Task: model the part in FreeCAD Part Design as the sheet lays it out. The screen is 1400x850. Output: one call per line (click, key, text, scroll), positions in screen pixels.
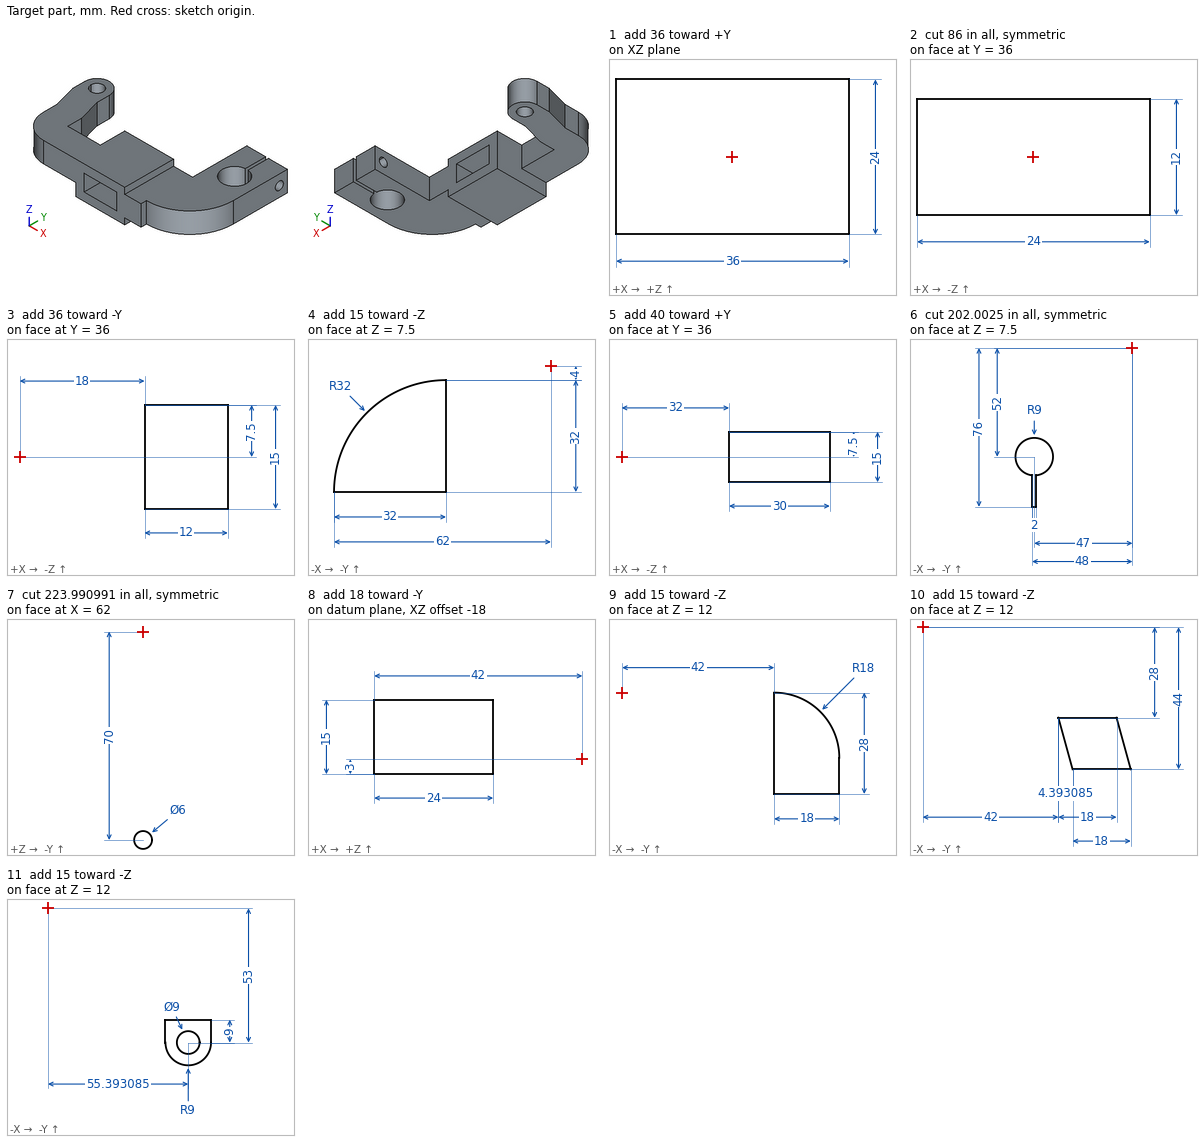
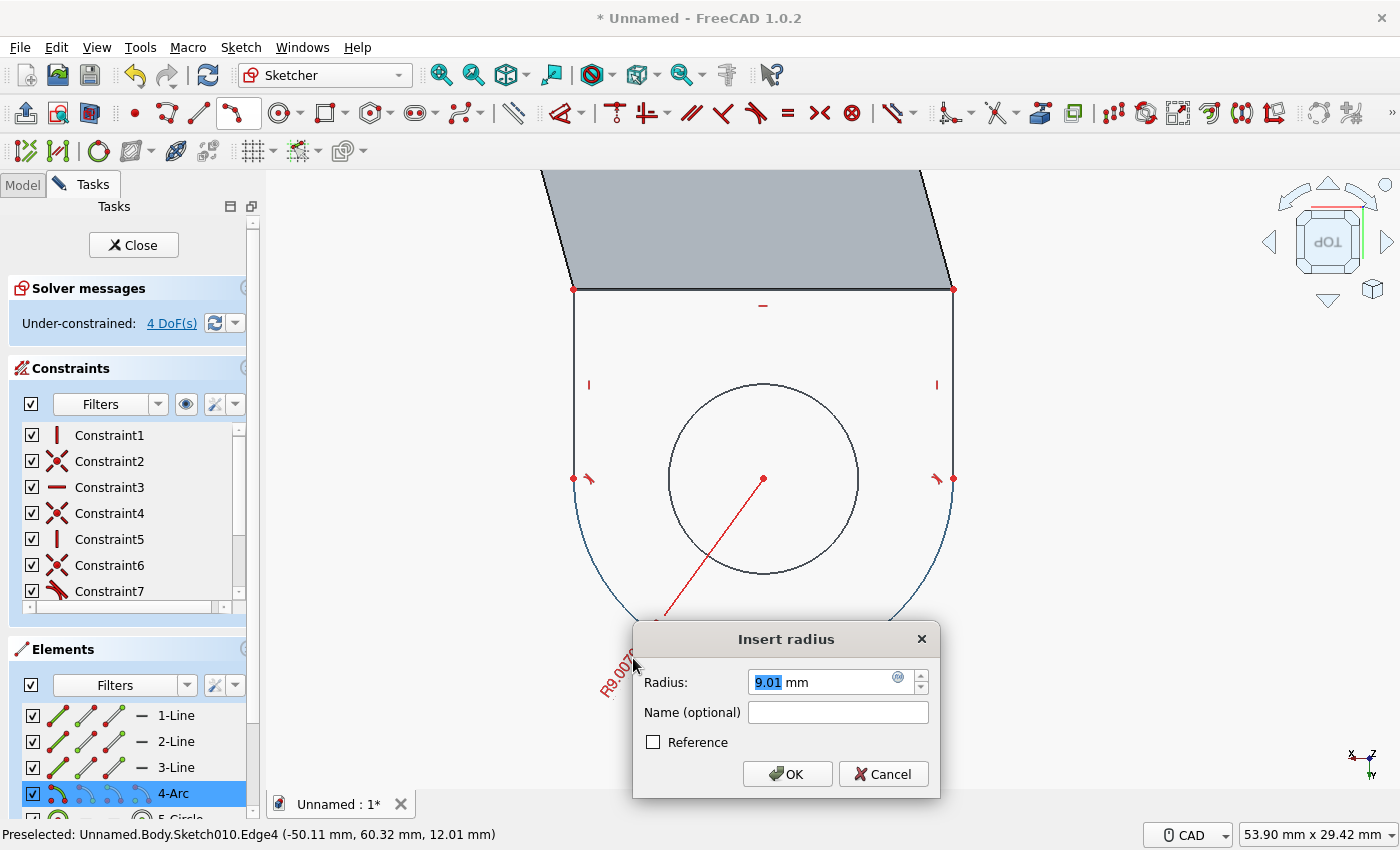
text(9)
key(Return)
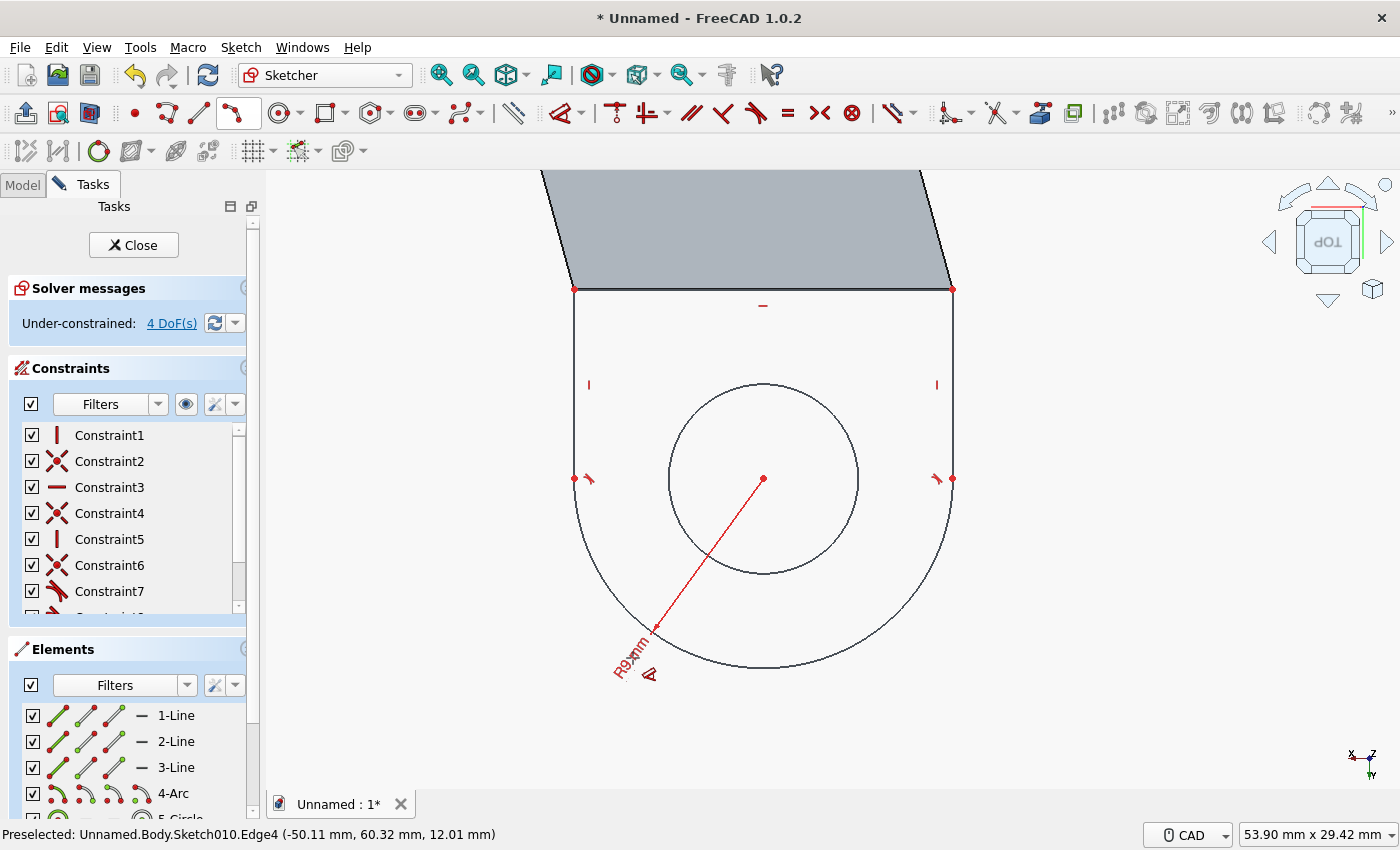
click(830, 412)
click(853, 389)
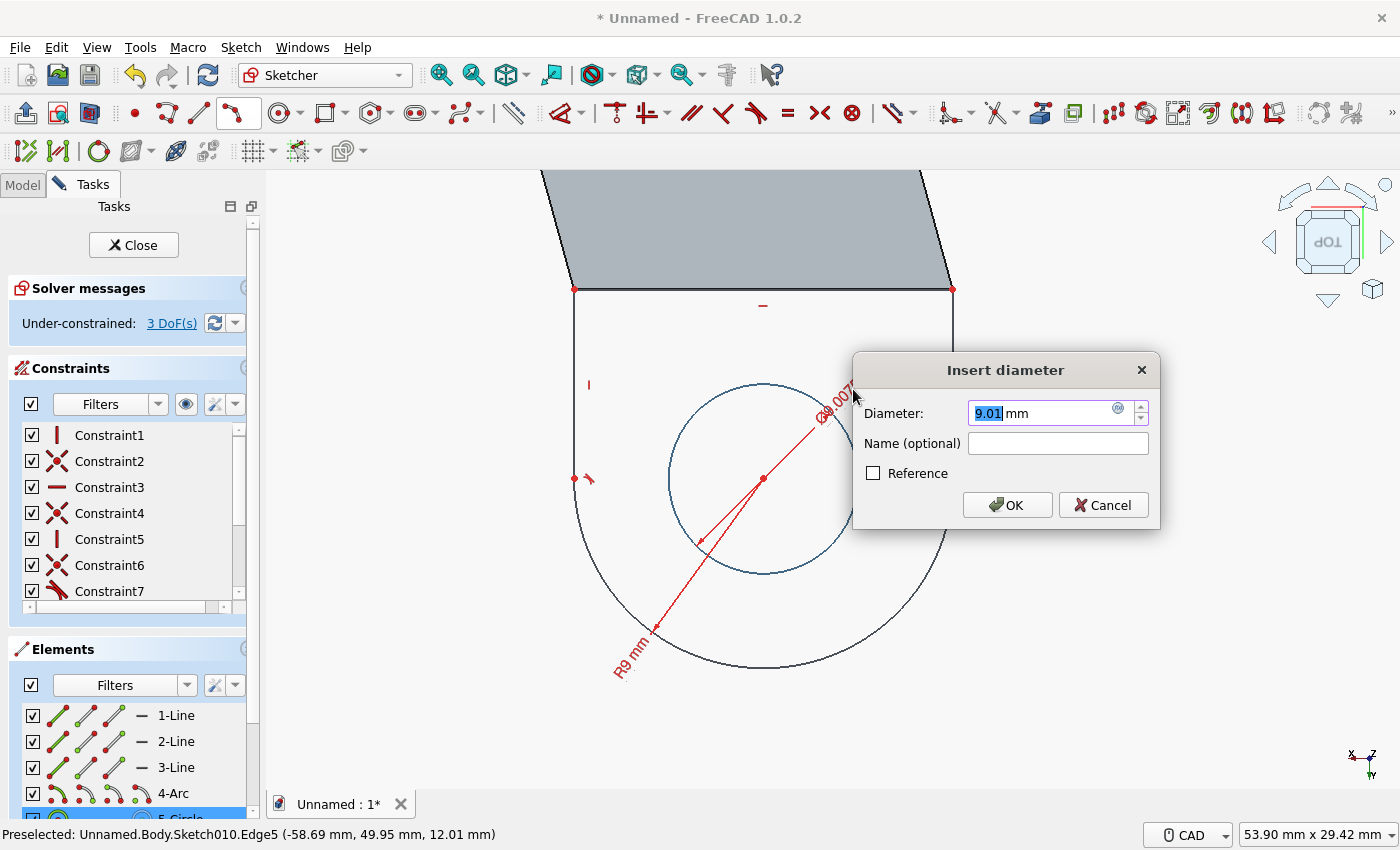
text(9)
key(Return)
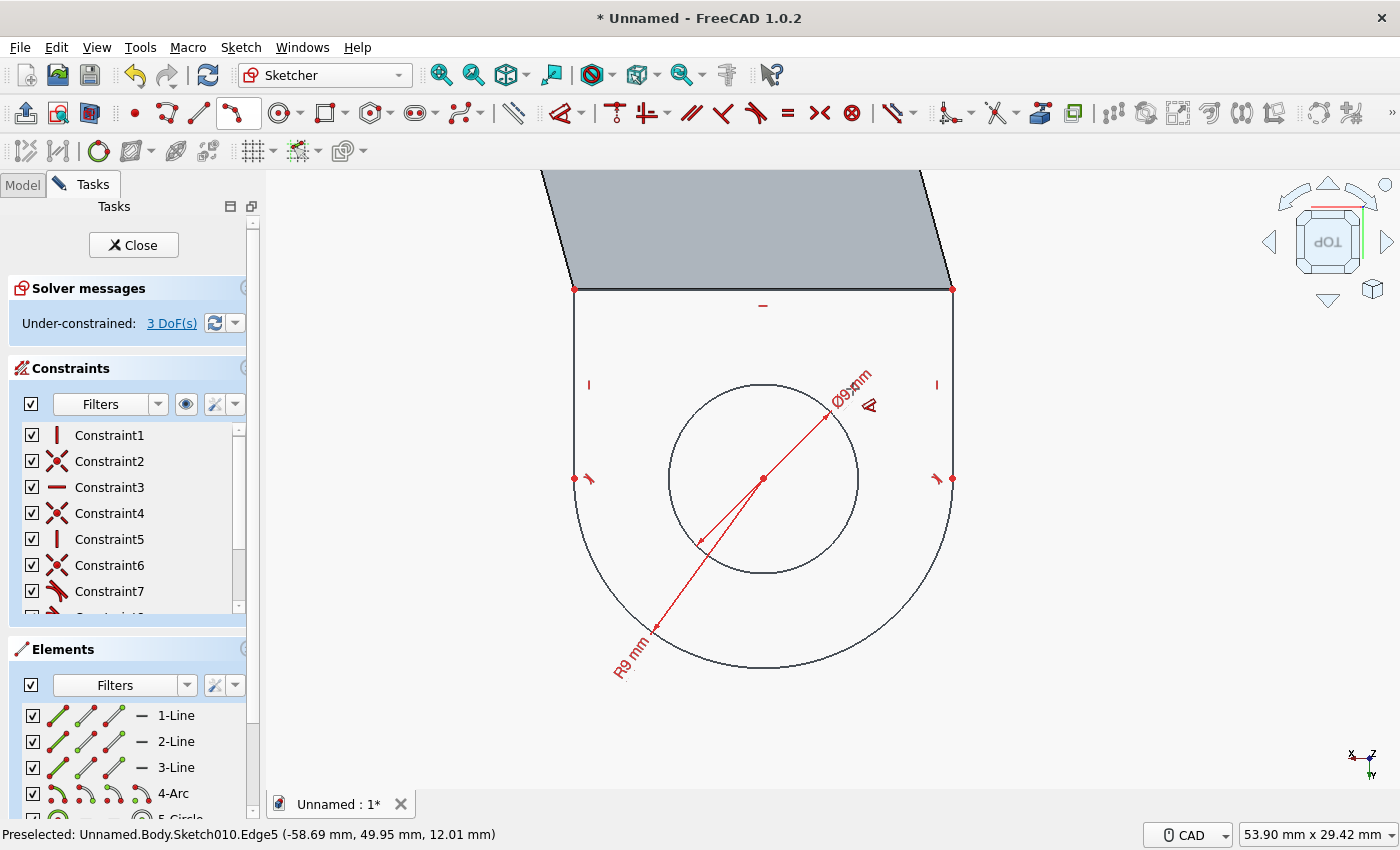
click(953, 422)
click(987, 384)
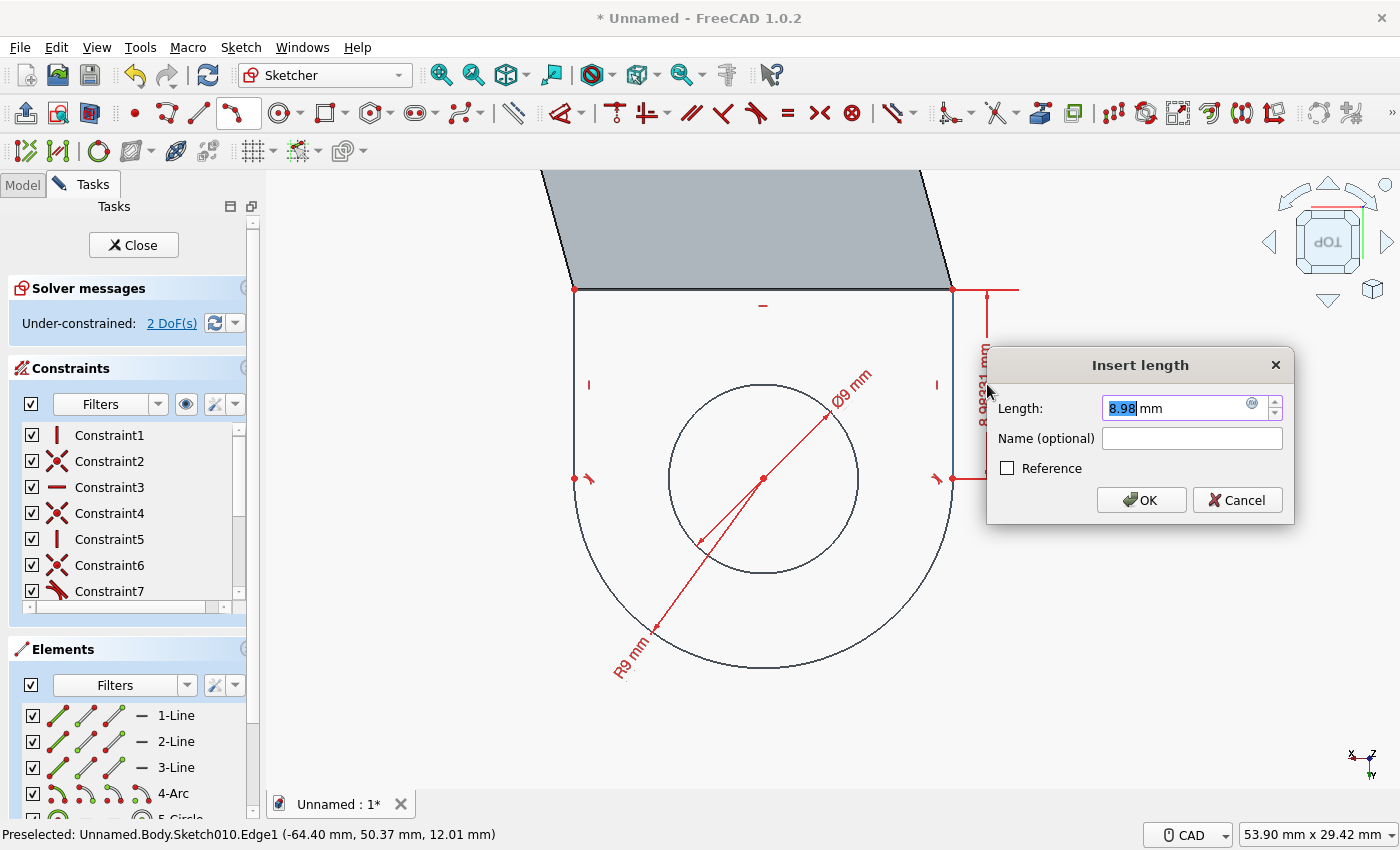
text(9)
key(Return)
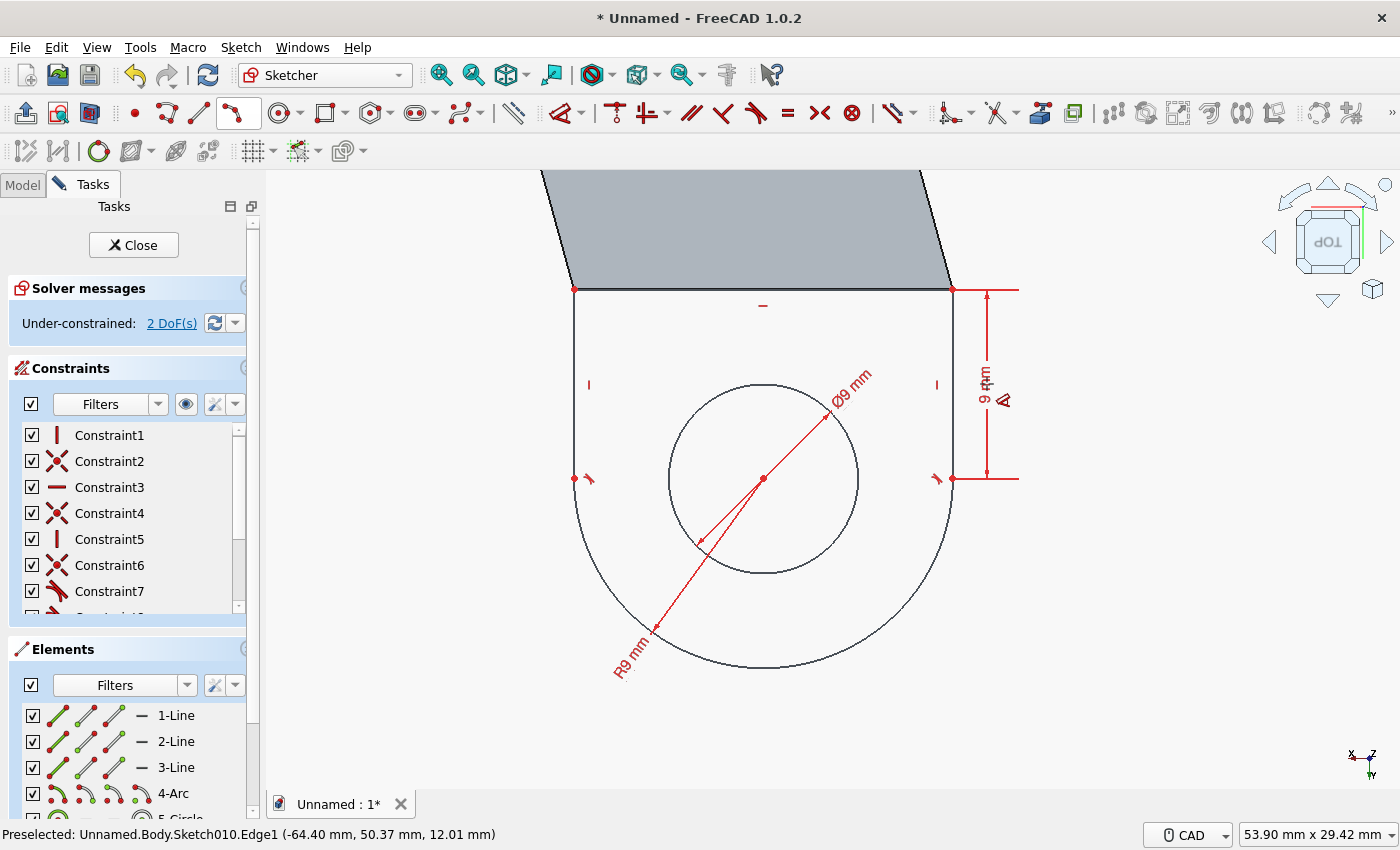
click(764, 479)
click(798, 338)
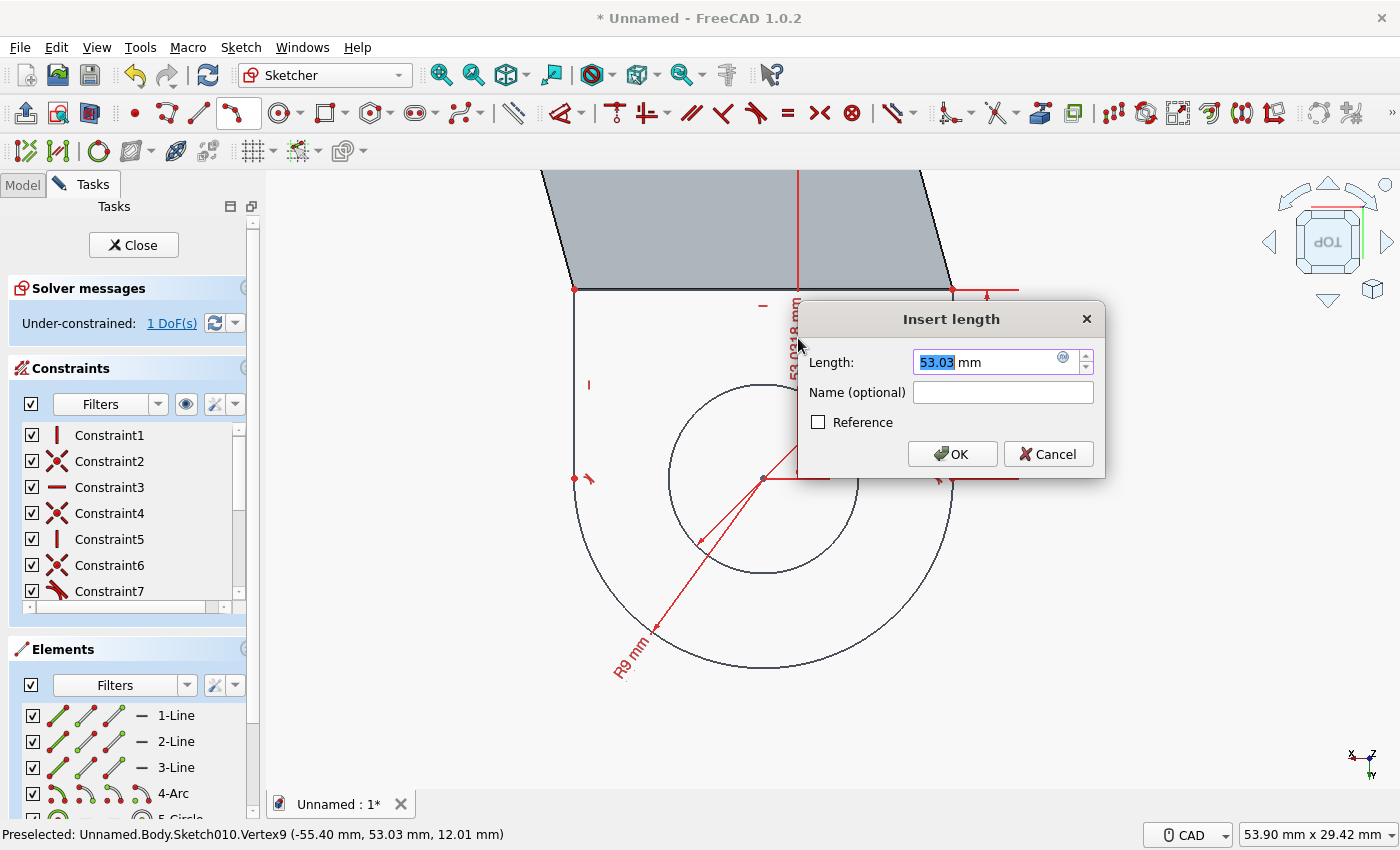
text(53)
key(Return)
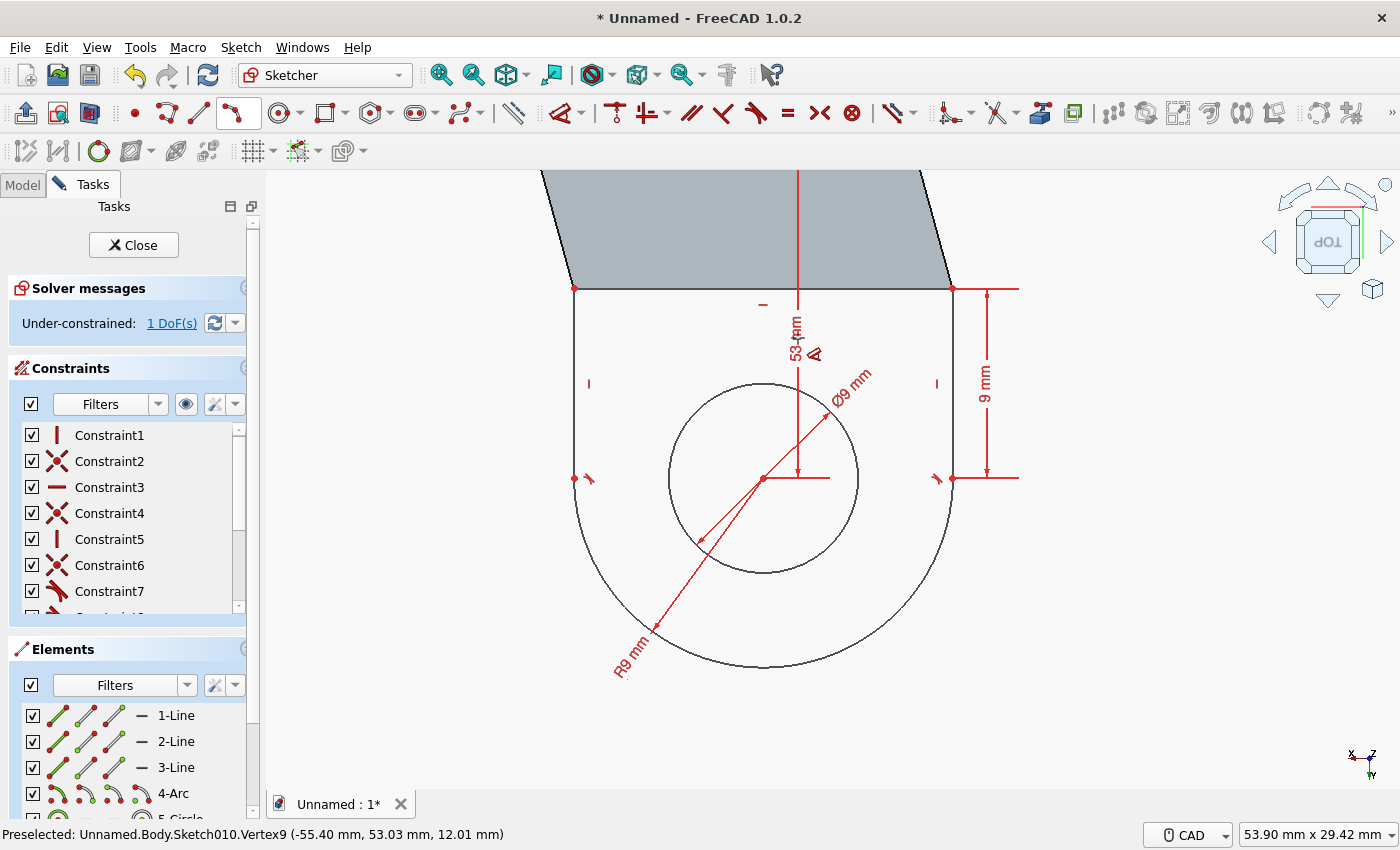
click(764, 478)
click(529, 512)